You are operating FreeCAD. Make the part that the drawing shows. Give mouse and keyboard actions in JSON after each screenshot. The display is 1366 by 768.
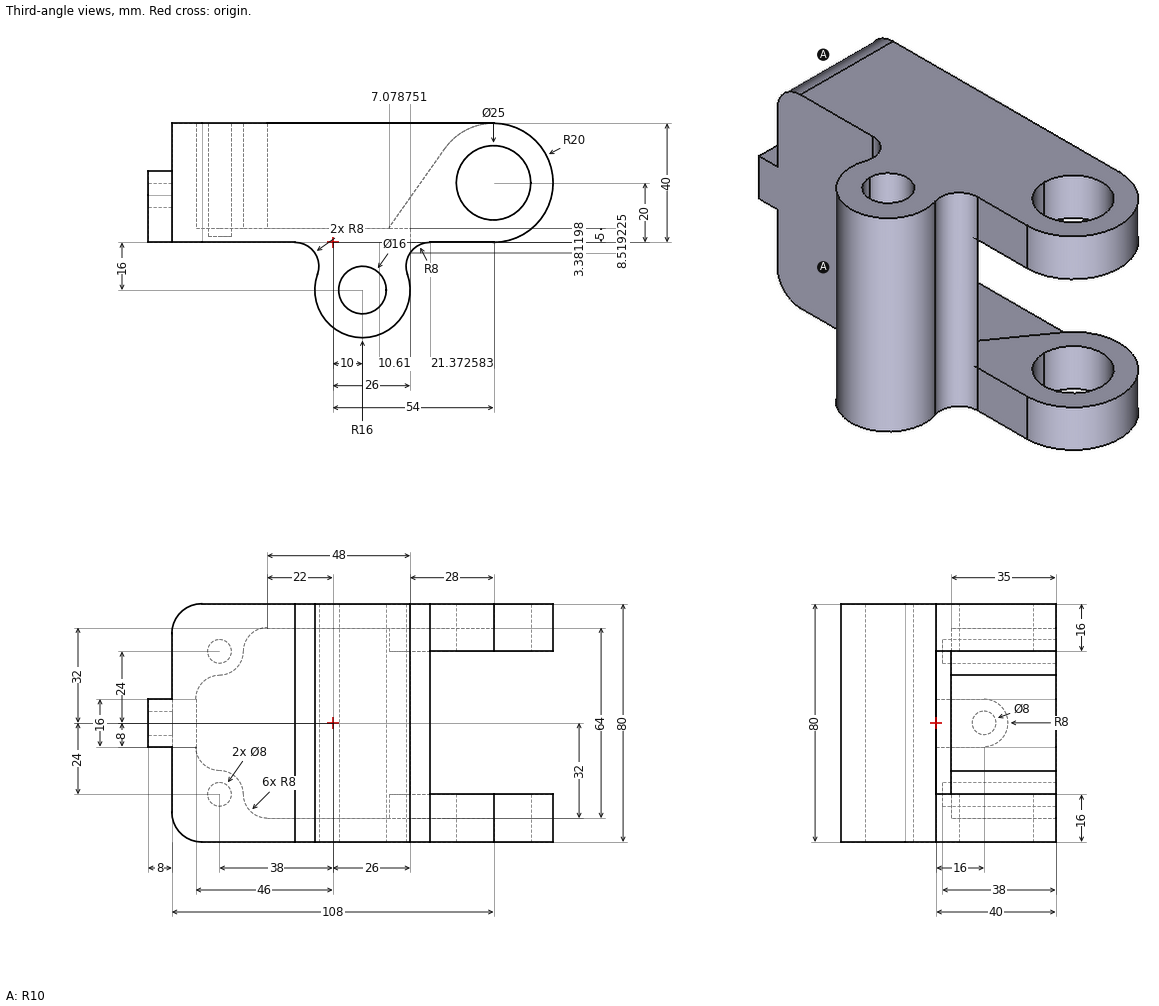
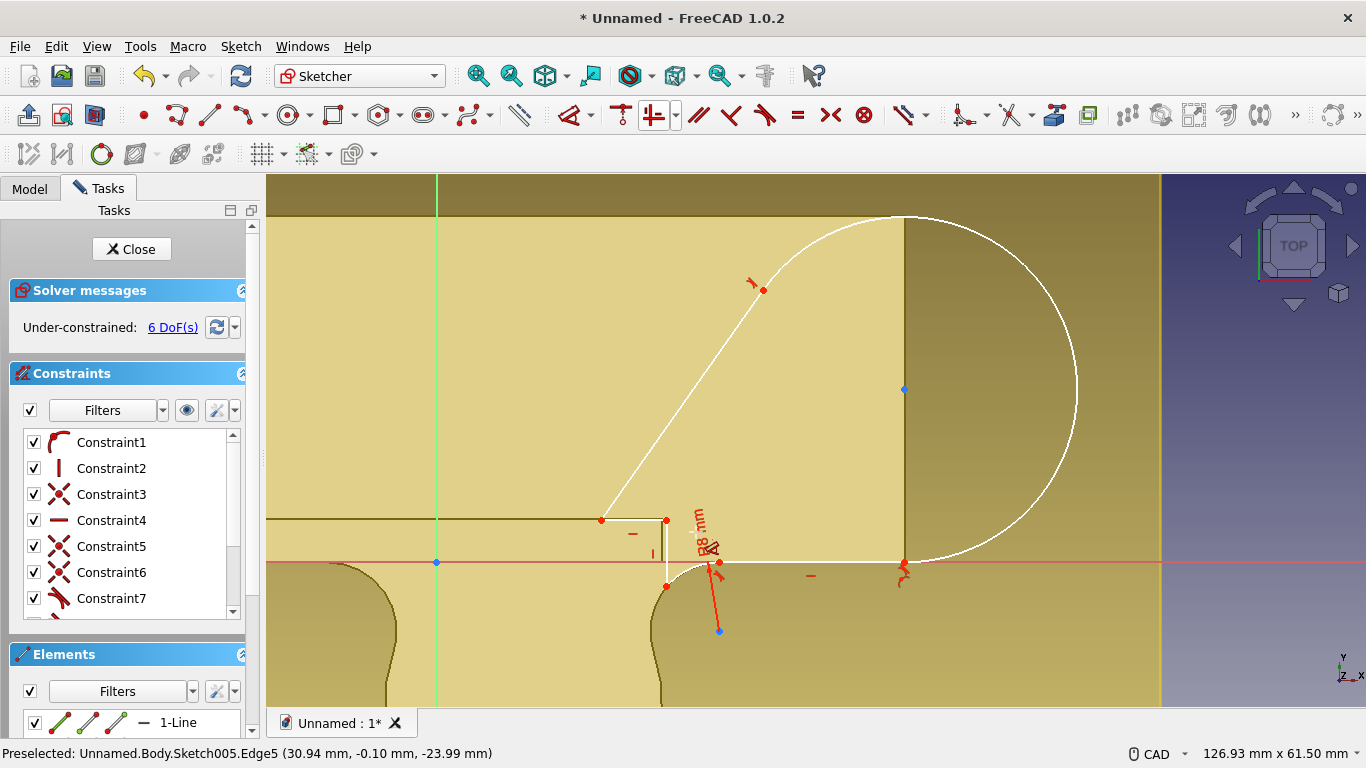
{"action": "left_click", "coordinate": [1067, 447]}
{"action": "left_click", "coordinate": [1097, 458]}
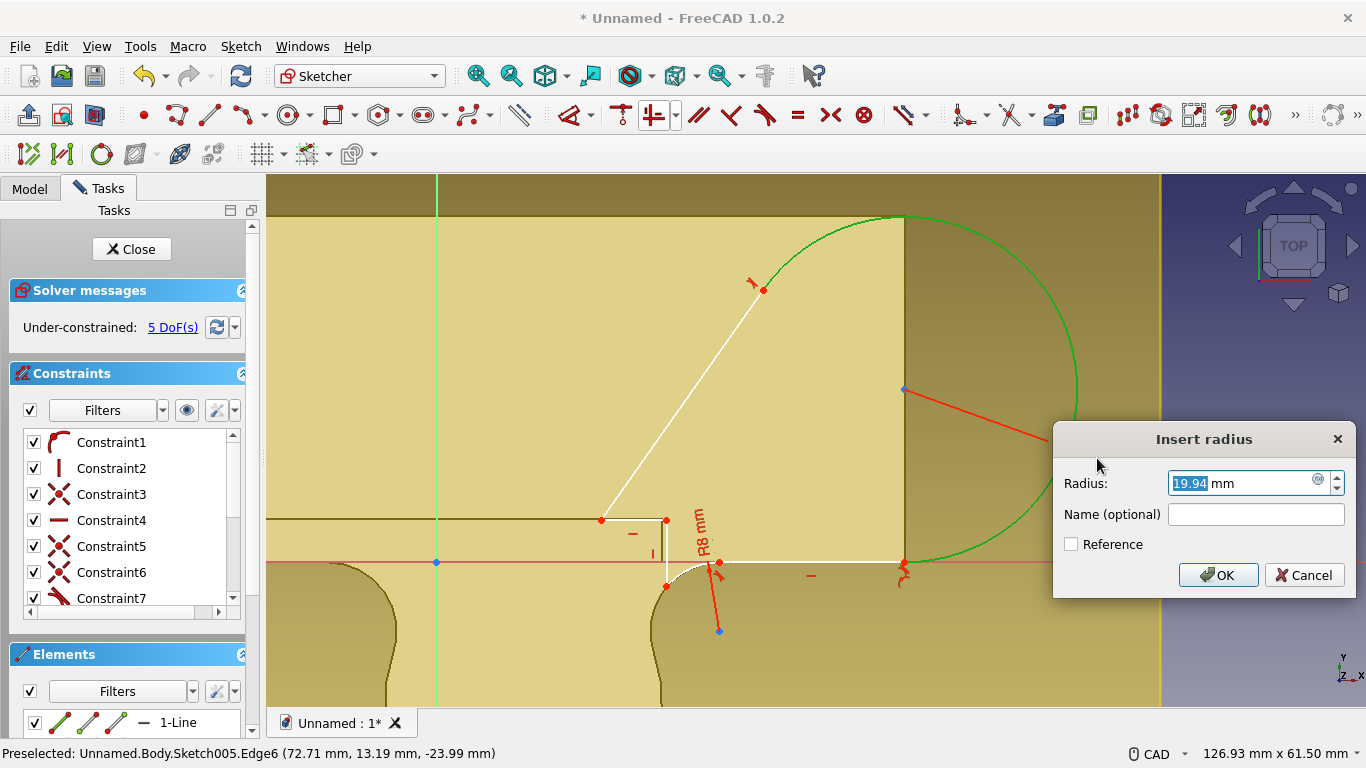
{"action": "type", "text": "20"}
{"action": "key", "text": "Return"}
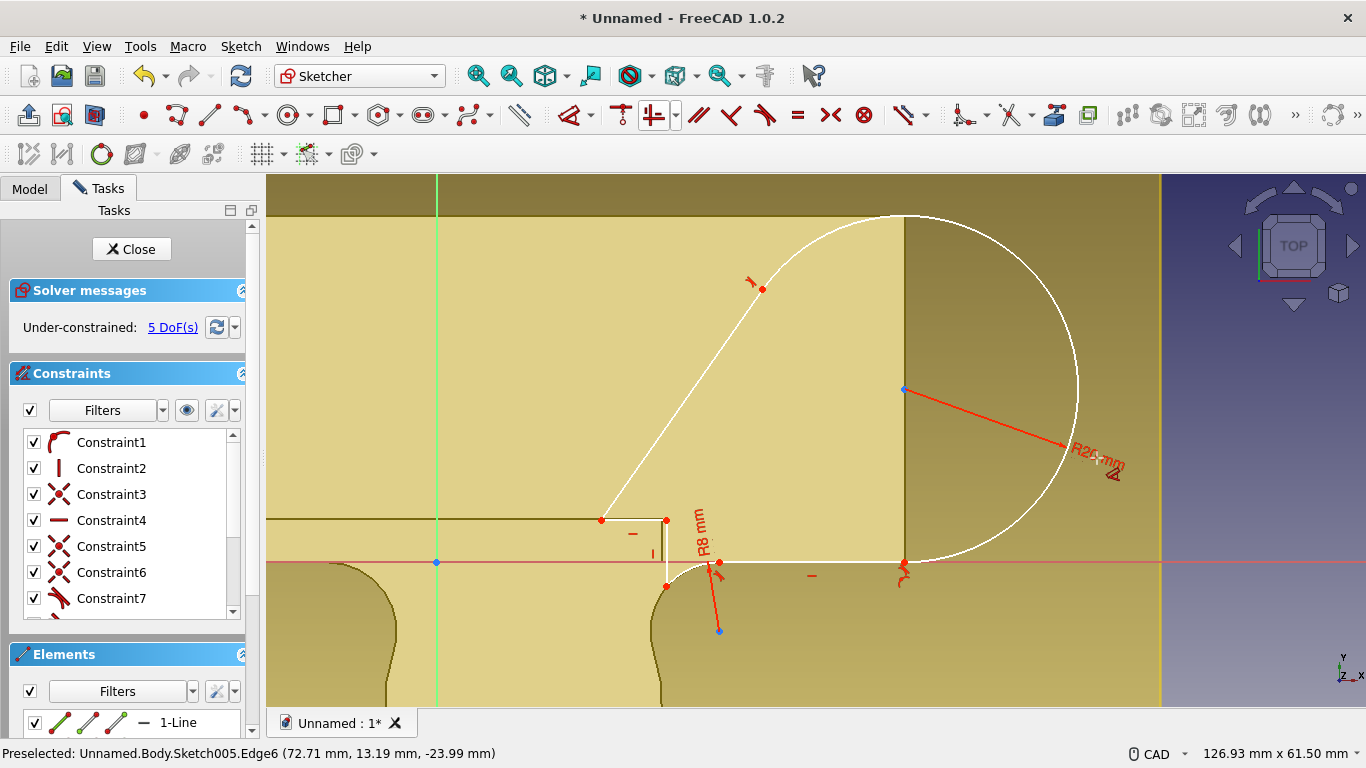
{"action": "left_click", "coordinate": [667, 520]}
{"action": "left_click", "coordinate": [403, 541]}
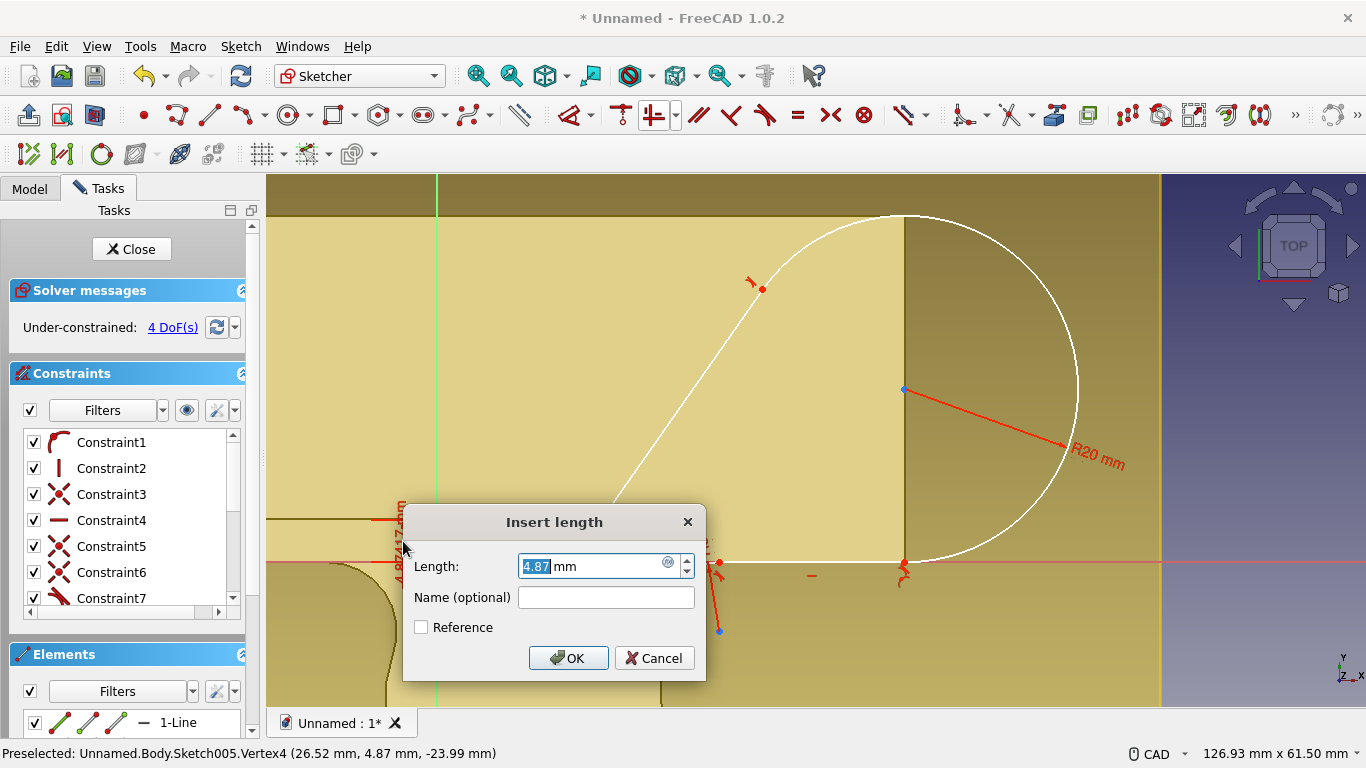
{"action": "type", "text": "5"}
{"action": "key", "text": "Return"}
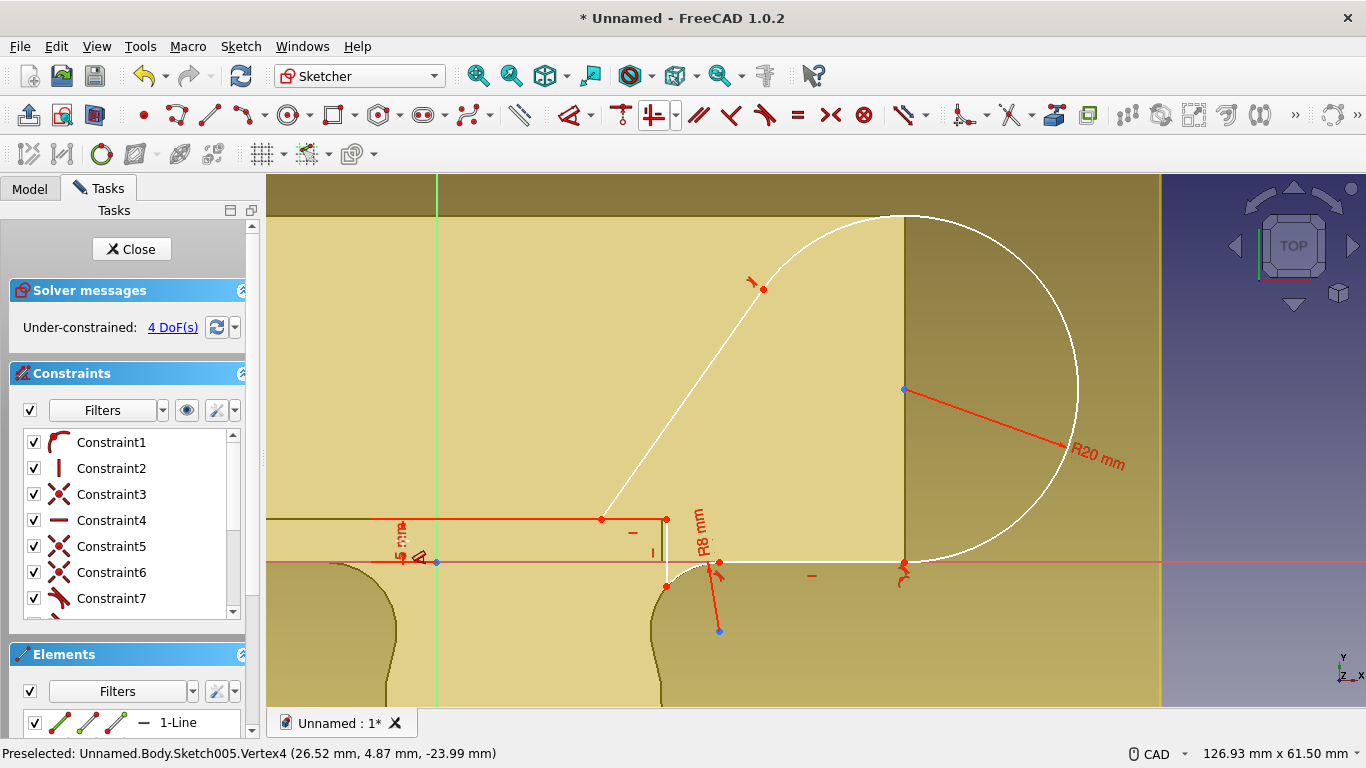
{"action": "left_click", "coordinate": [905, 562]}
{"action": "left_click", "coordinate": [563, 596]}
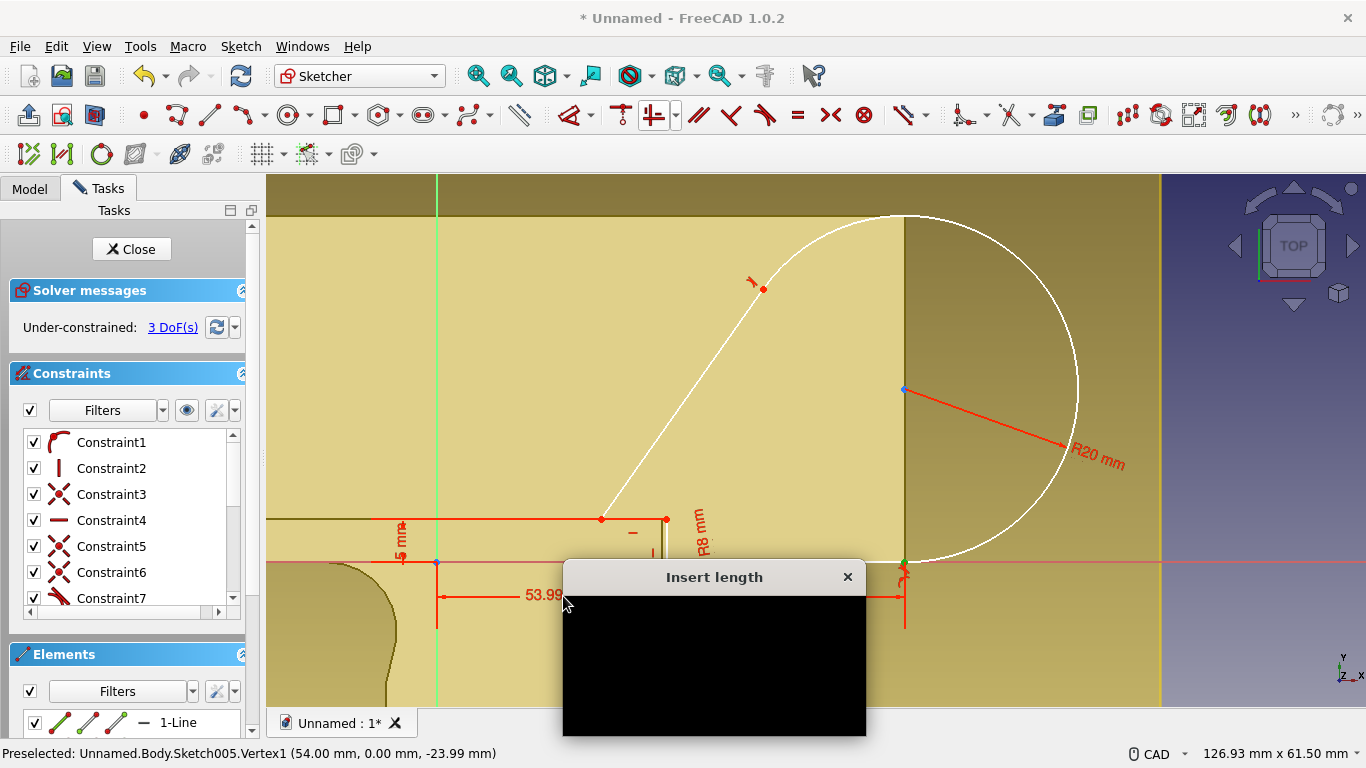
{"action": "type", "text": "54"}
{"action": "key", "text": "Return"}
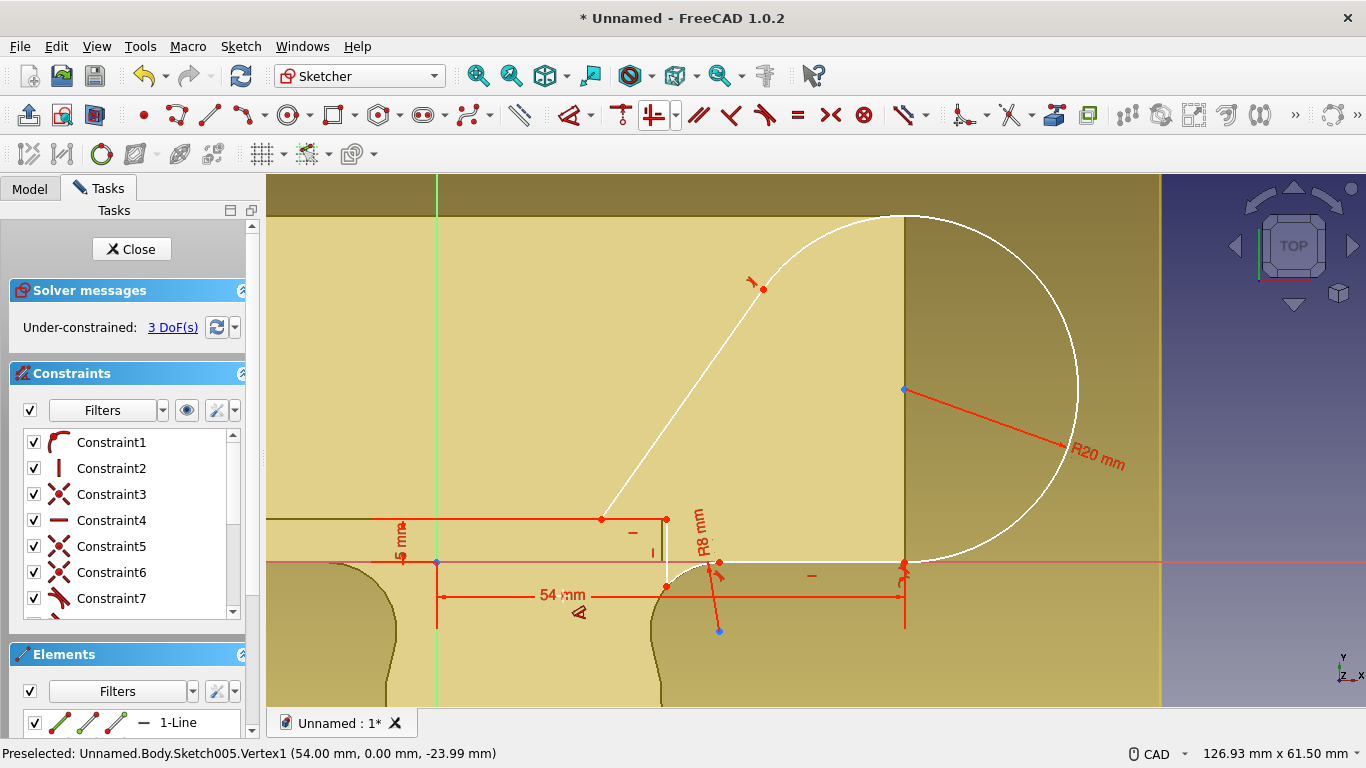
{"action": "left_click", "coordinate": [667, 587]}
{"action": "left_click", "coordinate": [552, 621]}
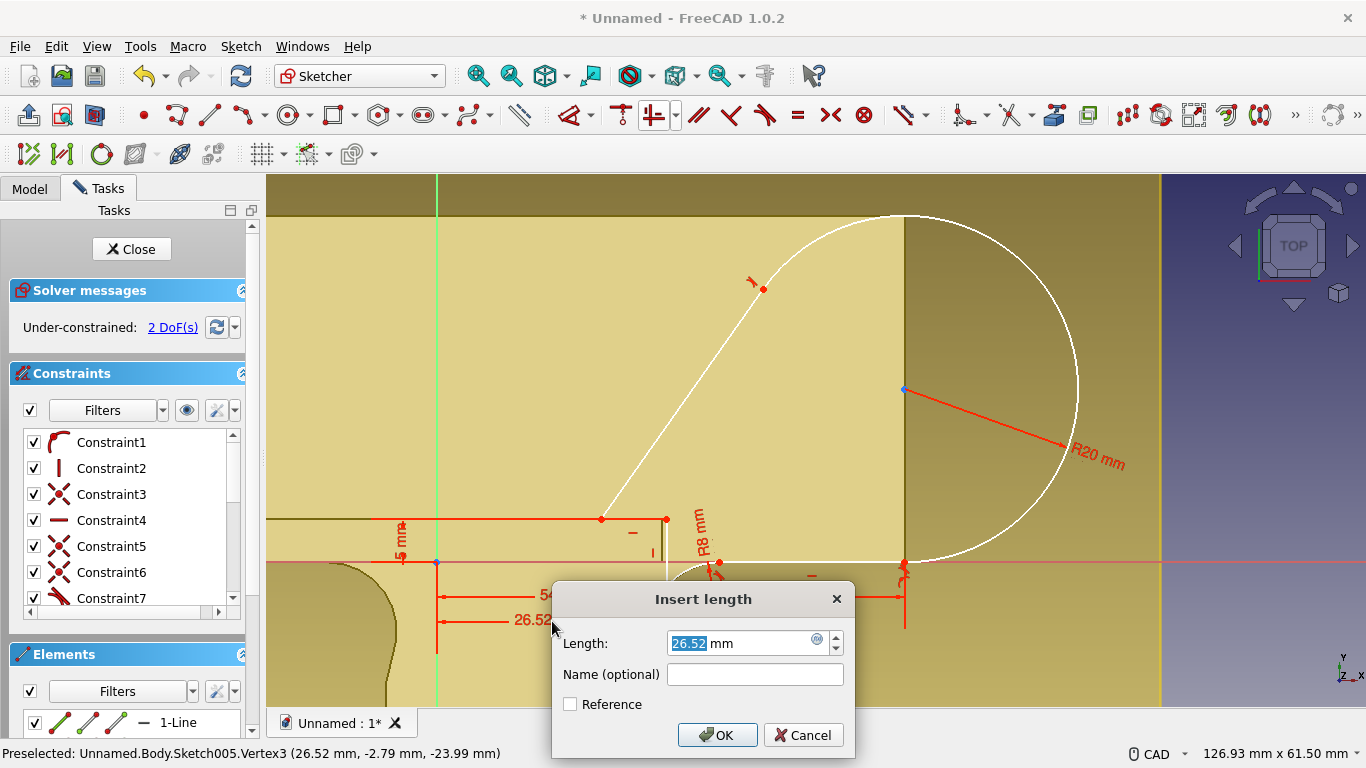
{"action": "type", "text": "26"}
{"action": "key", "text": "Return"}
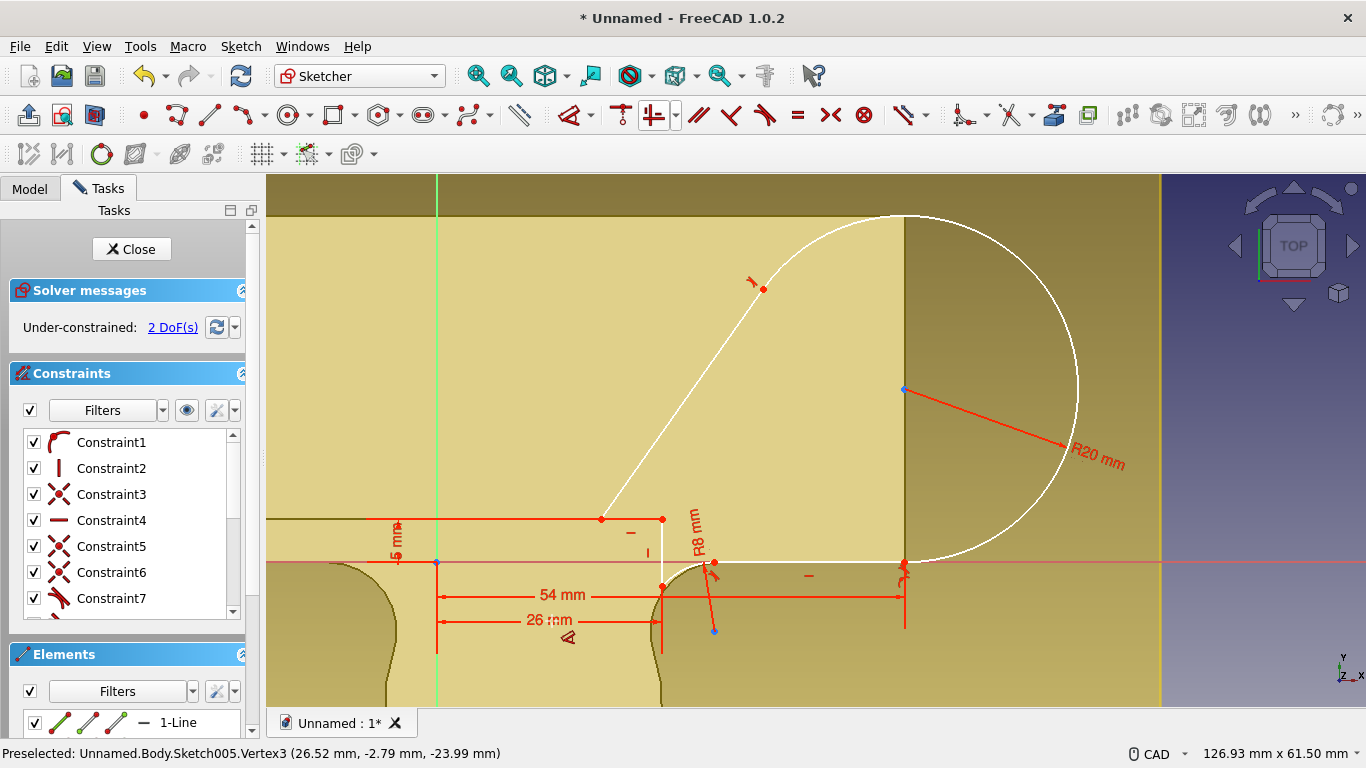
{"action": "left_click", "coordinate": [662, 566]}
{"action": "left_click", "coordinate": [604, 537]}